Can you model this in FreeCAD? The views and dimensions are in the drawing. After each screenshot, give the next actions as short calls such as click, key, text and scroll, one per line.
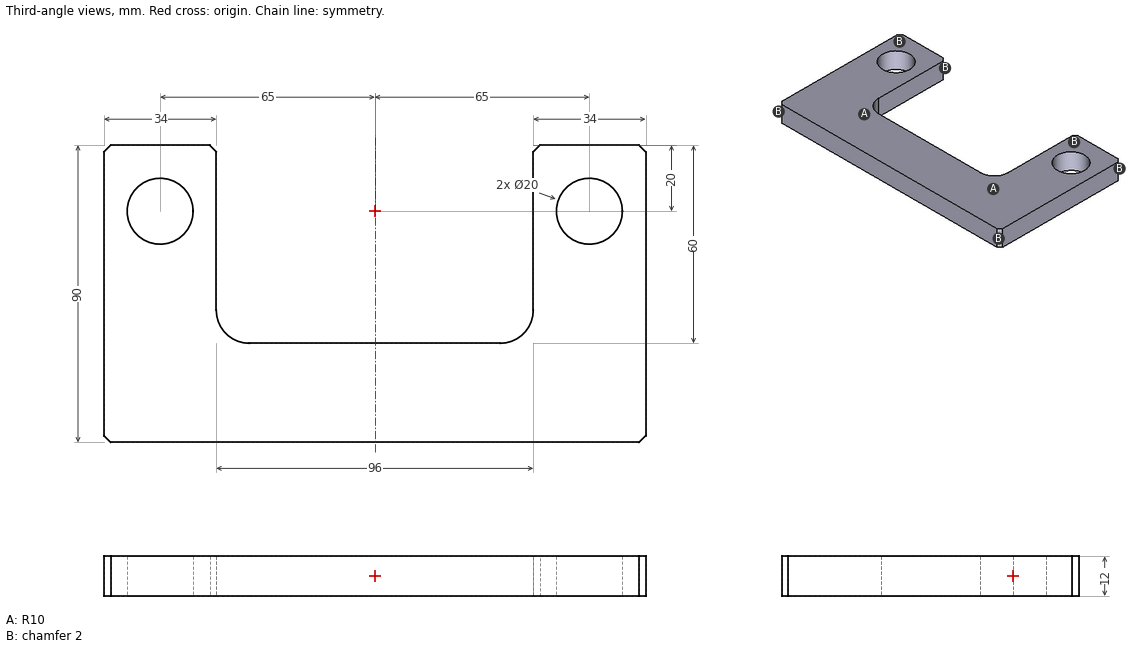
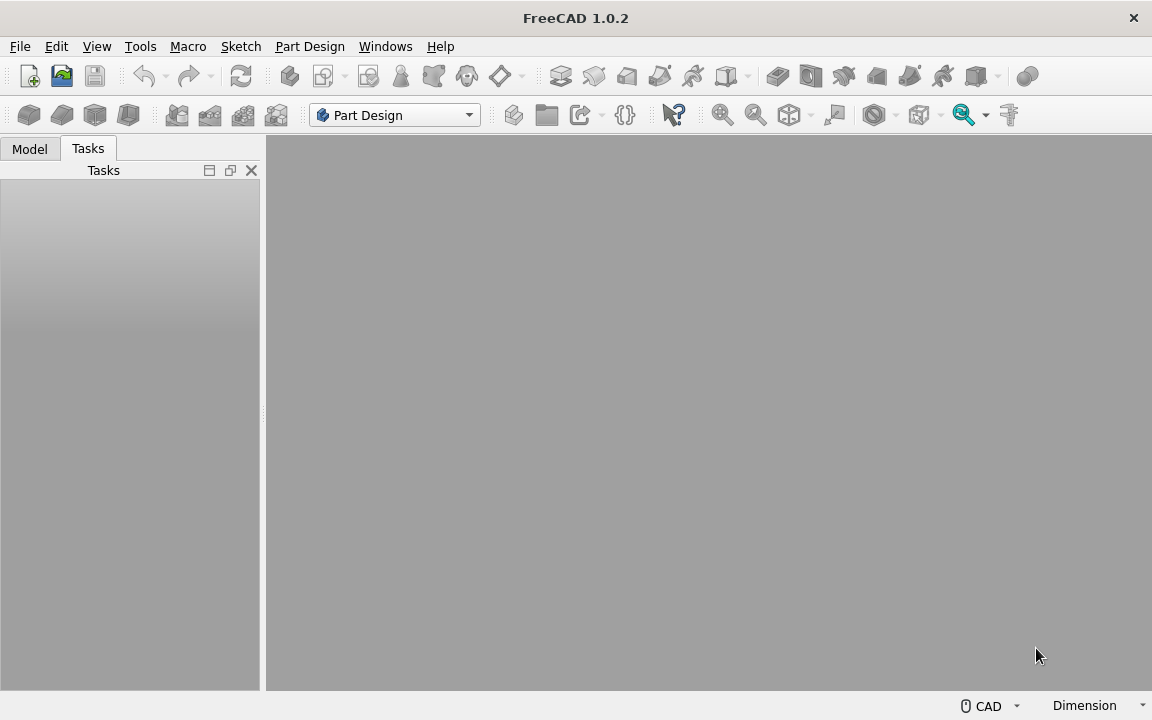
click(29, 76)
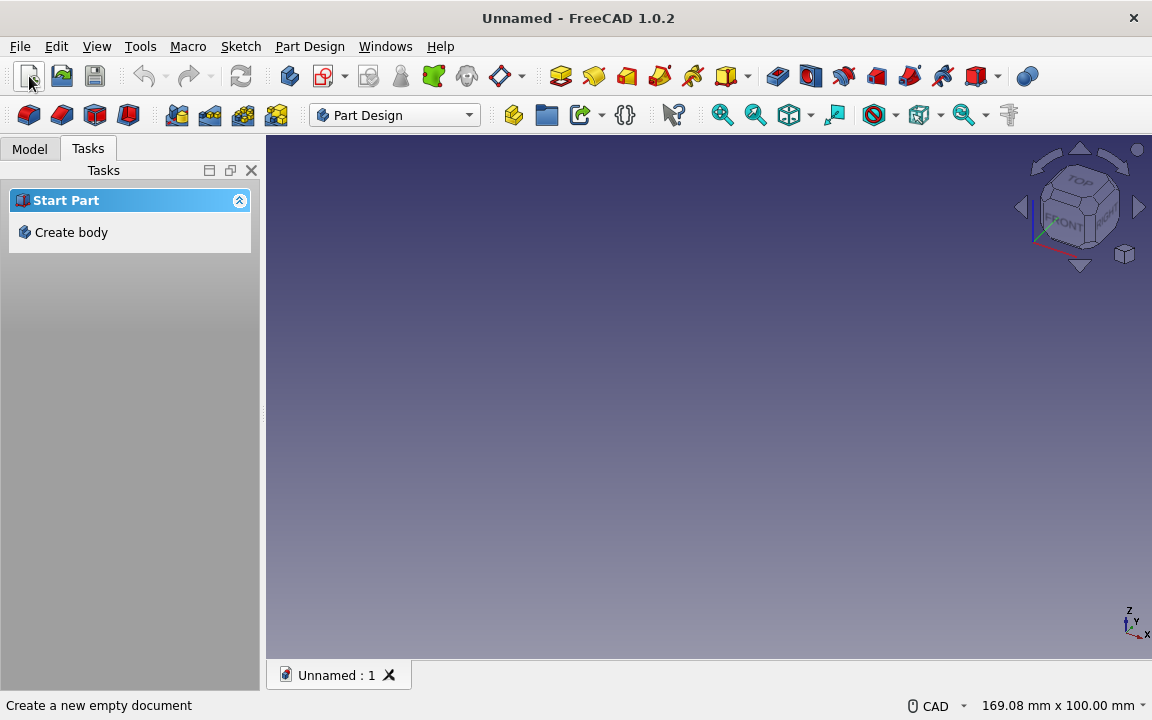
click(322, 76)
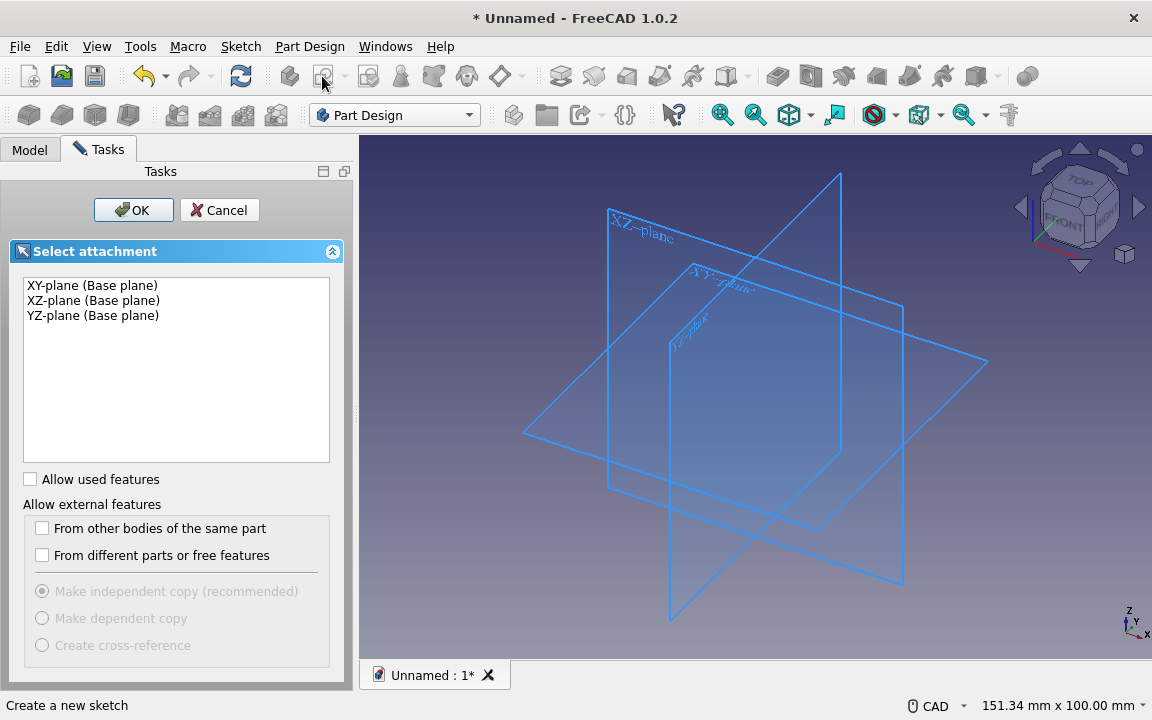
click(84, 286)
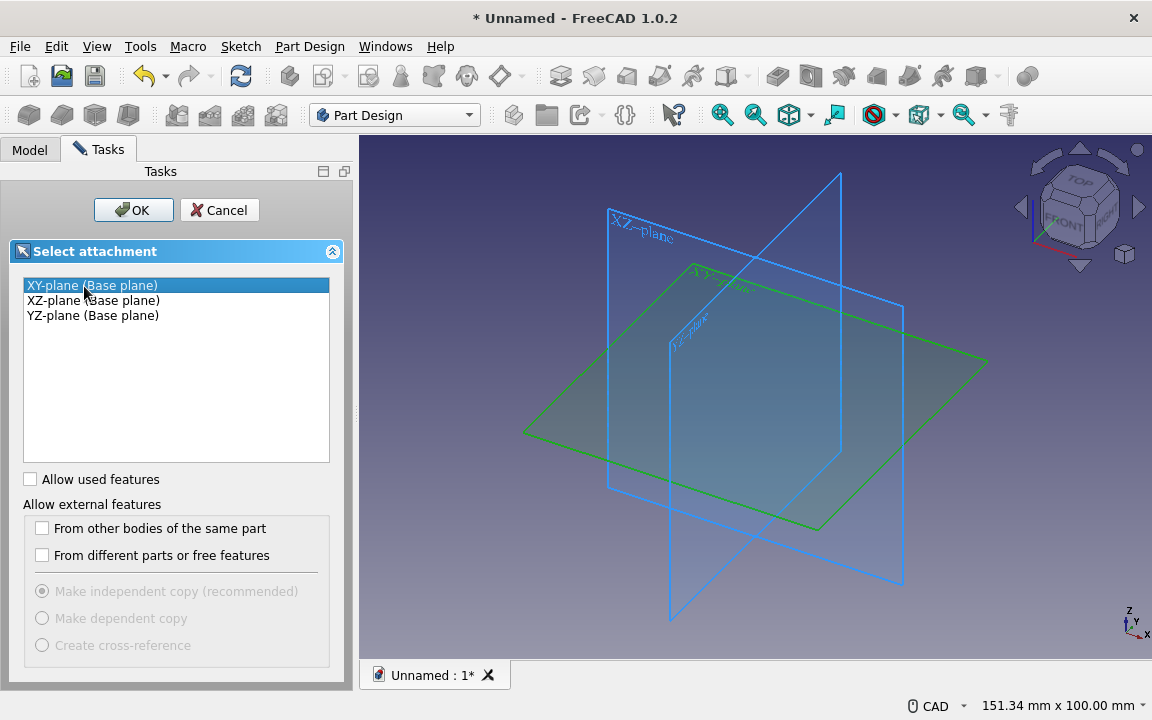
click(134, 210)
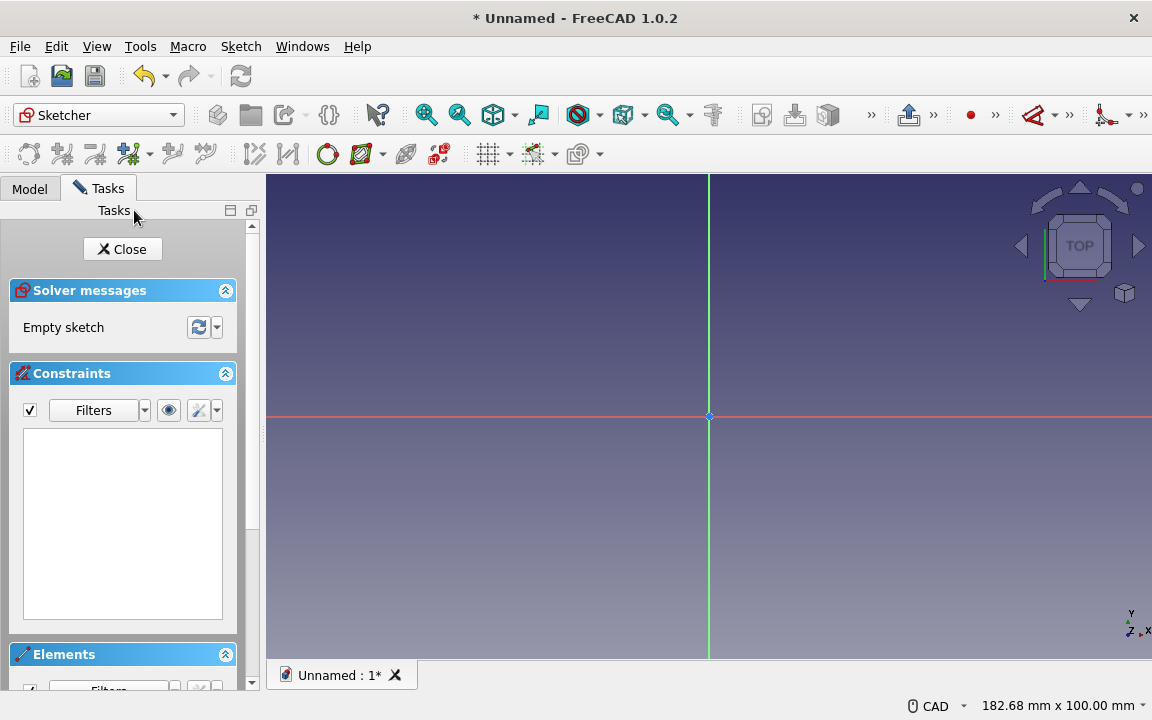
scroll(501, 202, down, 2)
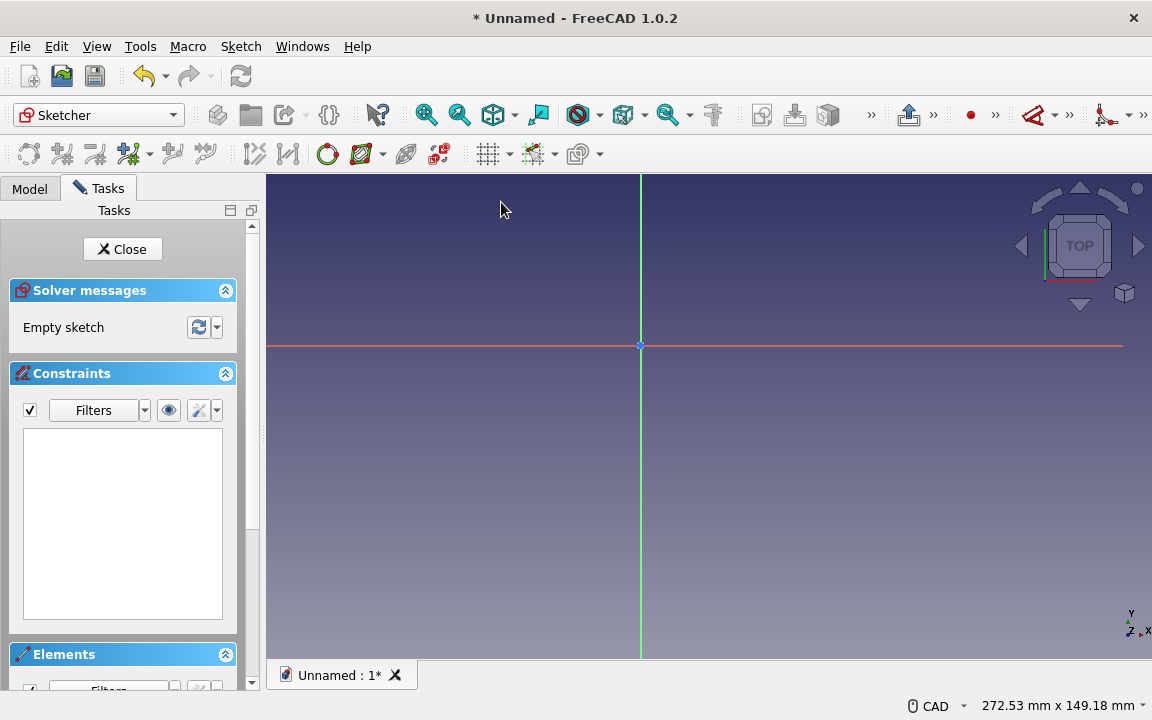
key(g)
key(m)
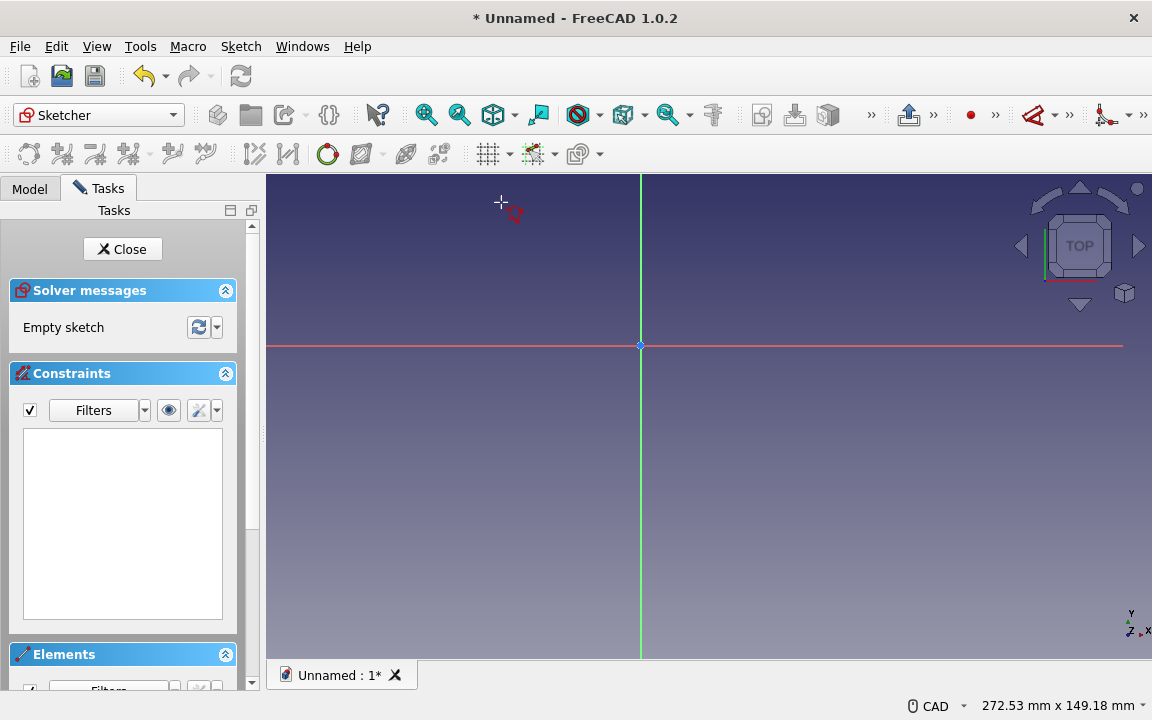
click(797, 281)
click(797, 476)
click(484, 476)
click(484, 281)
click(374, 281)
click(374, 573)
click(907, 573)
click(907, 281)
click(797, 282)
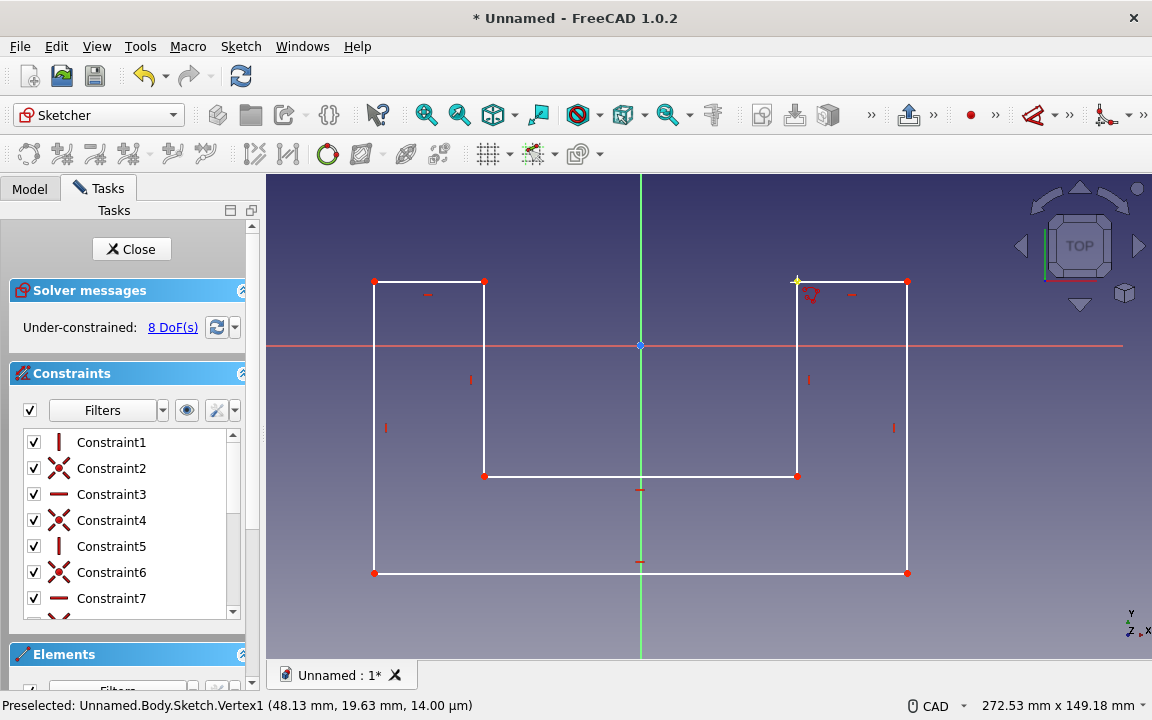
key(g)
key(c)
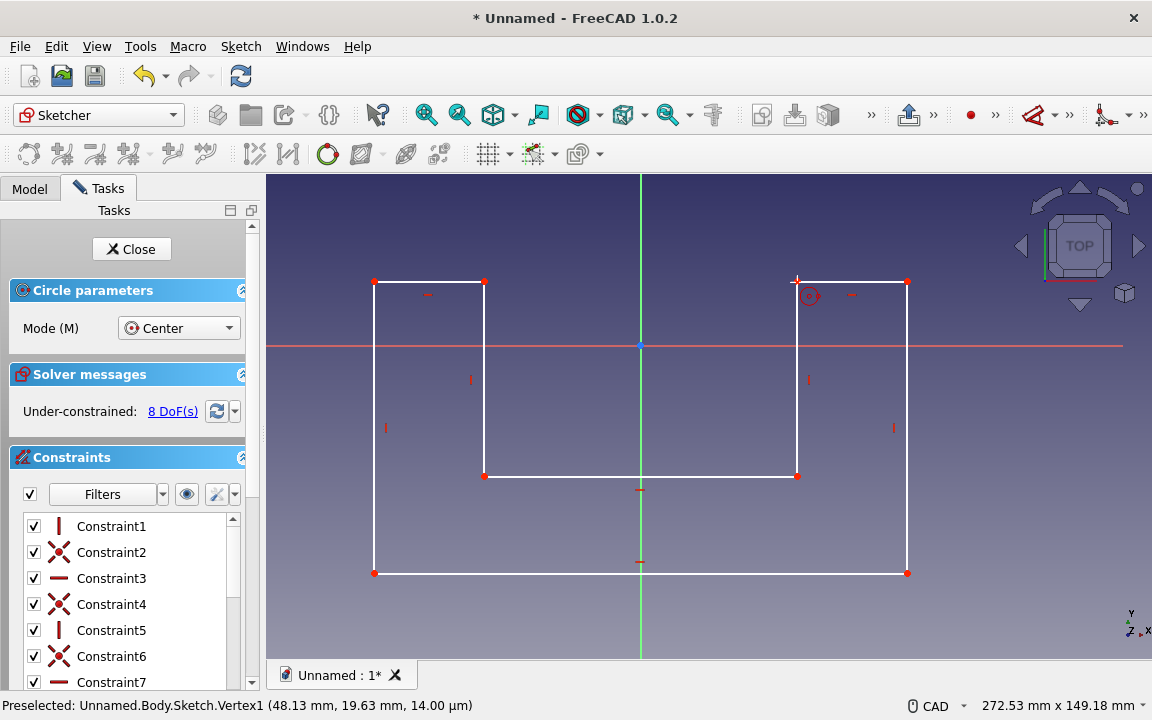
click(852, 346)
move(875, 323)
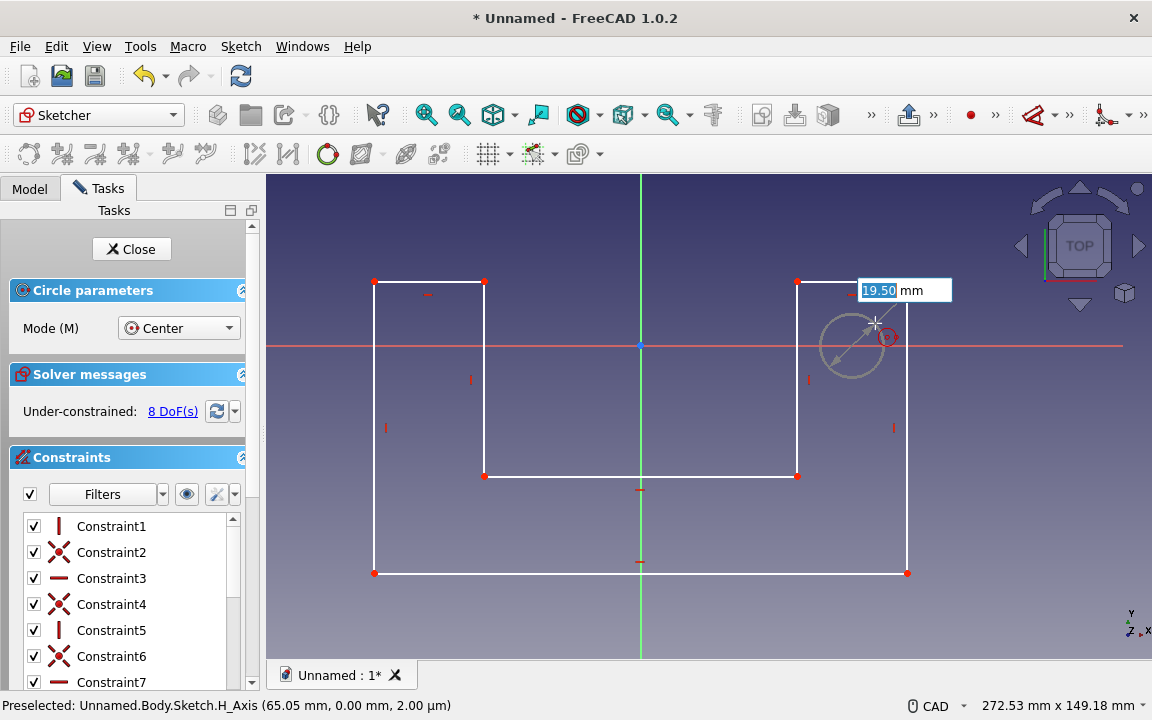
text(20)
key(Return)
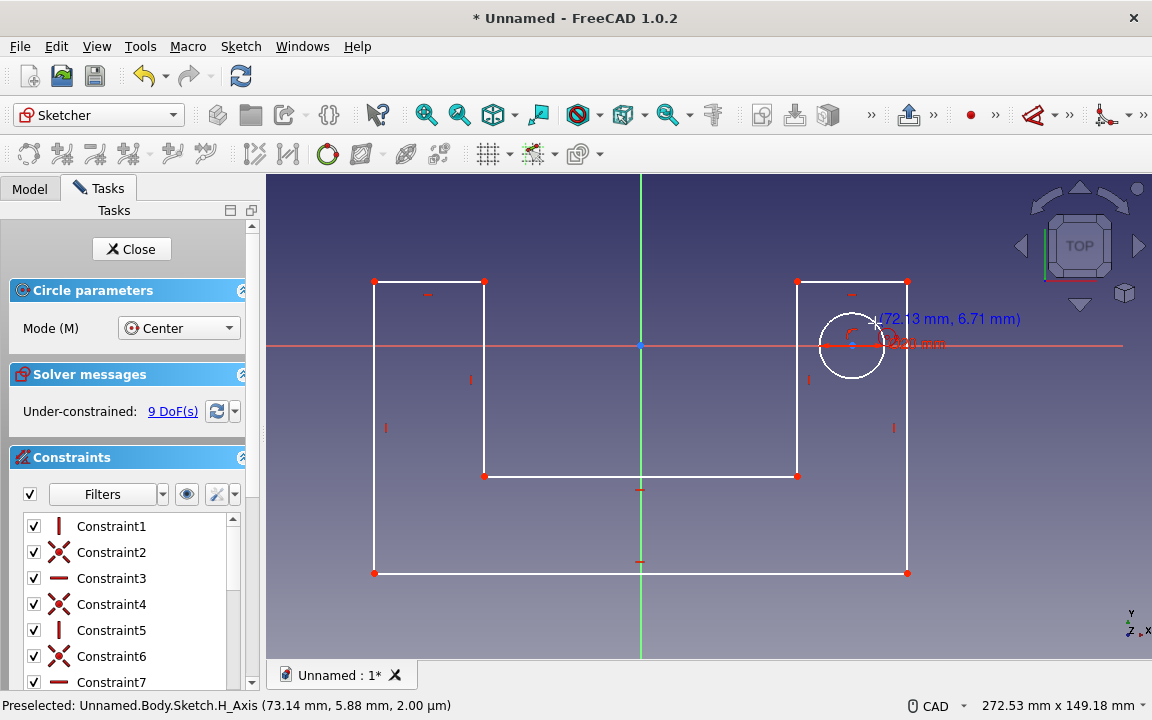
click(429, 346)
move(452, 323)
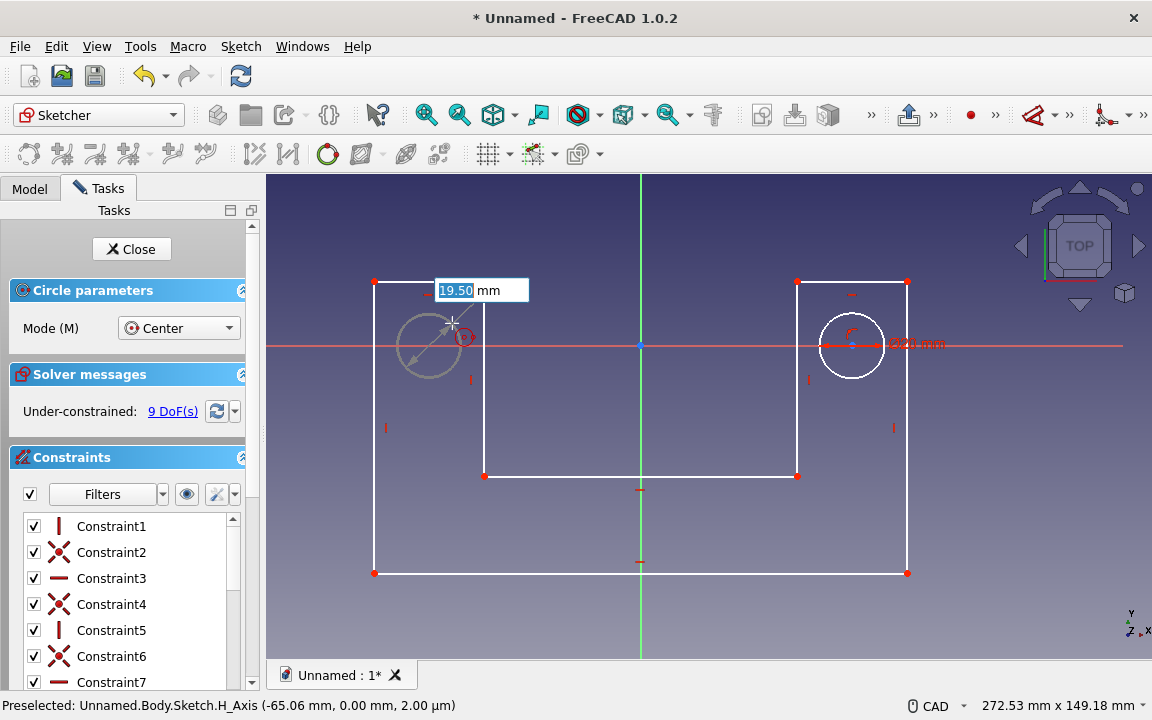
text(20)
key(Return)
key(Escape)